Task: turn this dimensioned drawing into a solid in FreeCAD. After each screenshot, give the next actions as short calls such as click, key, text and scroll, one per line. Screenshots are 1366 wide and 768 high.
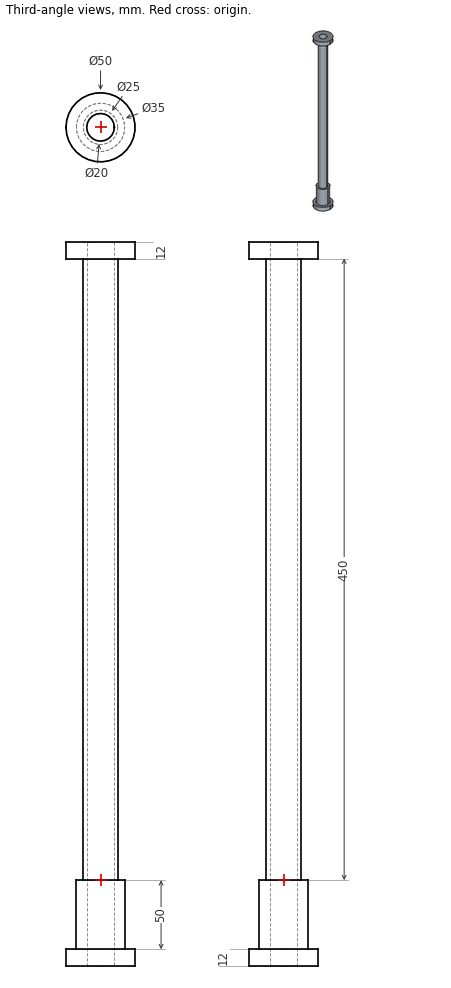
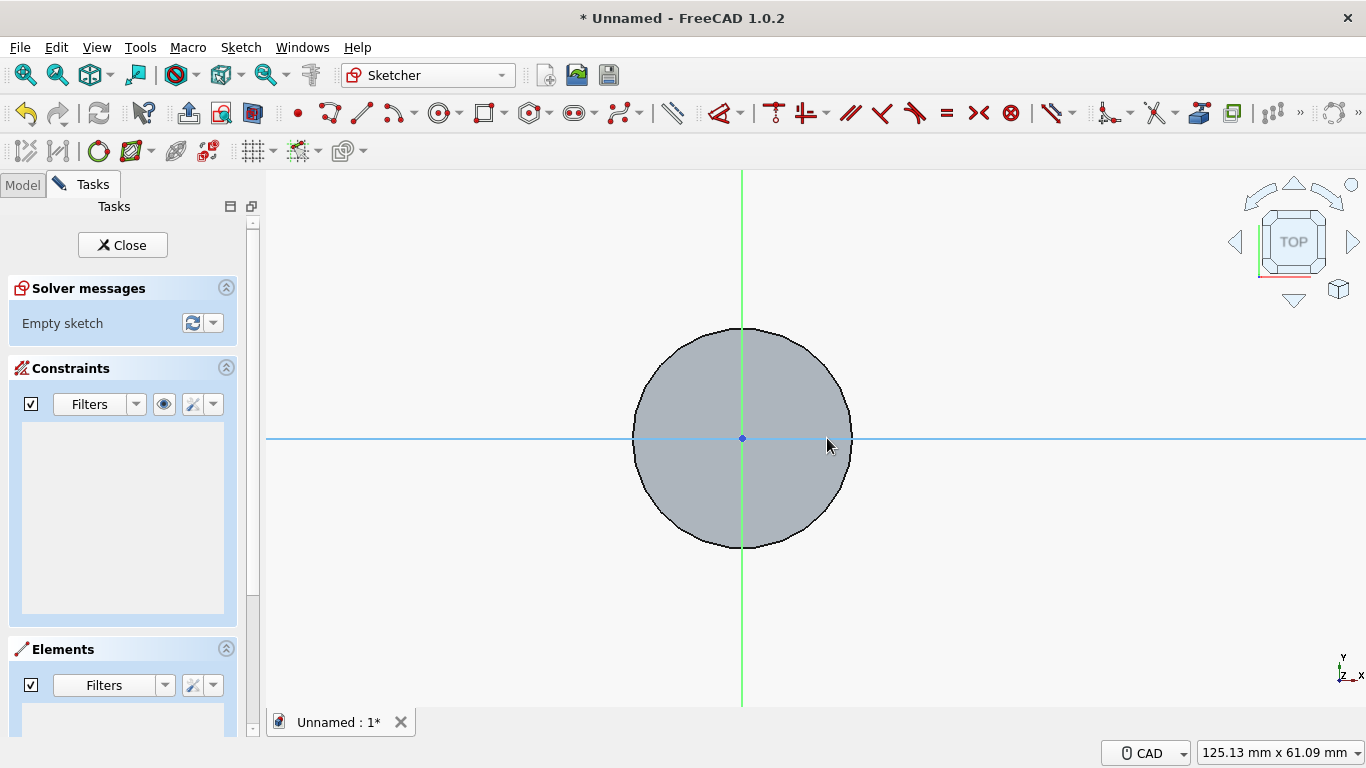
click(440, 114)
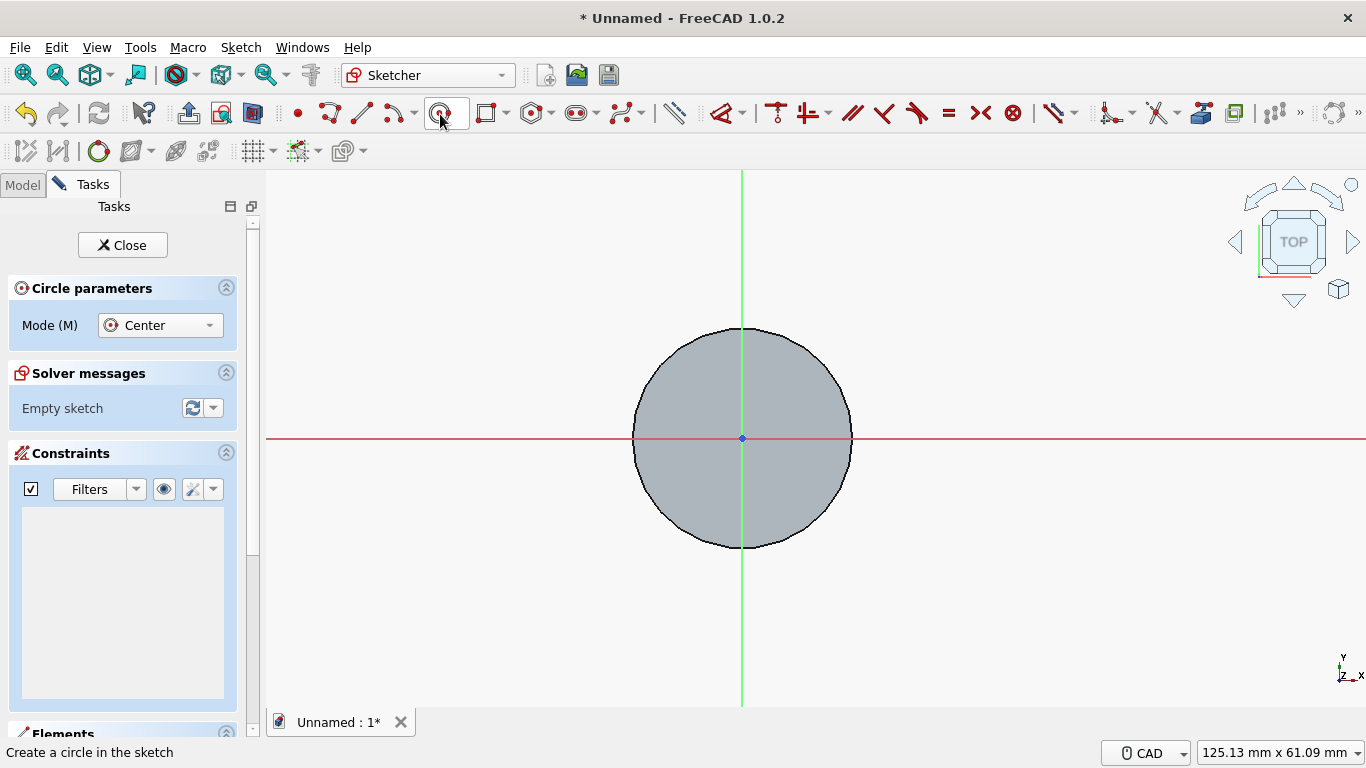
click(742, 438)
click(851, 330)
key(Escape)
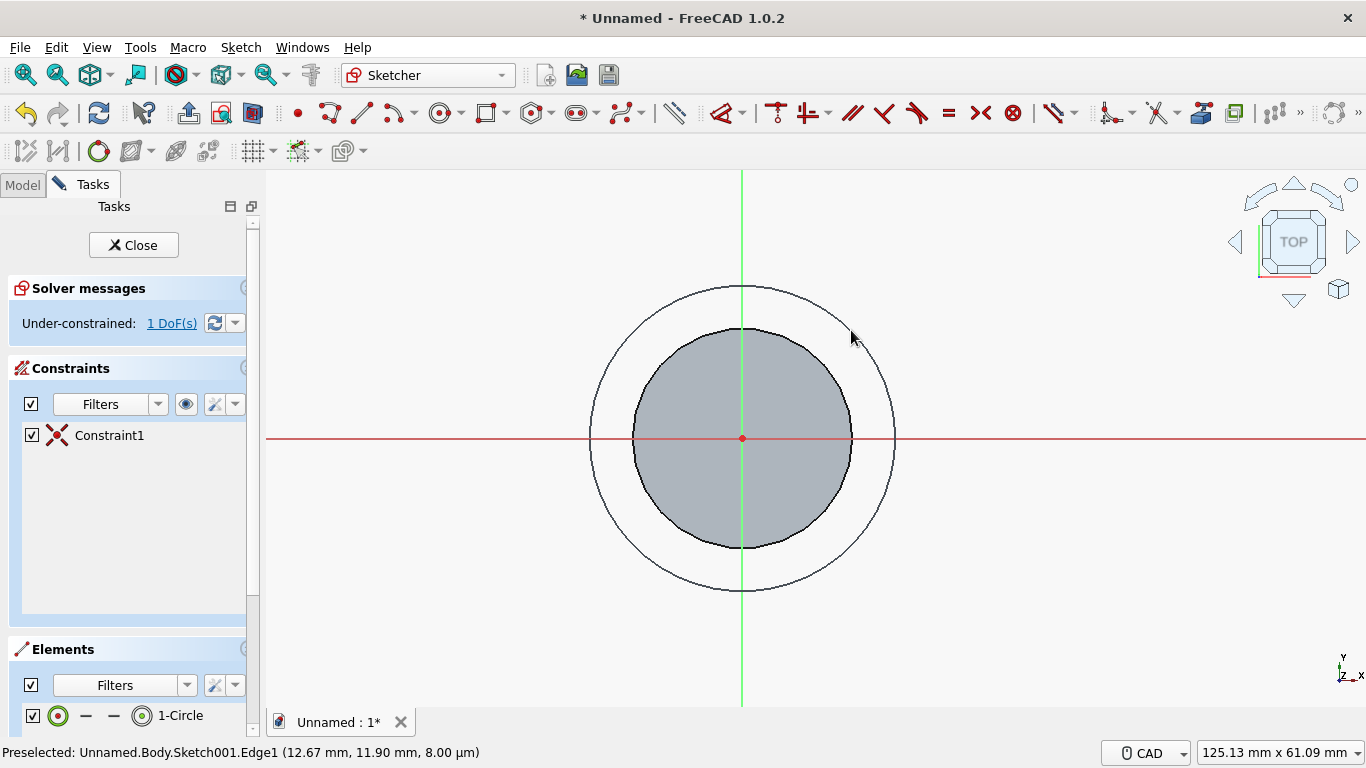
click(722, 114)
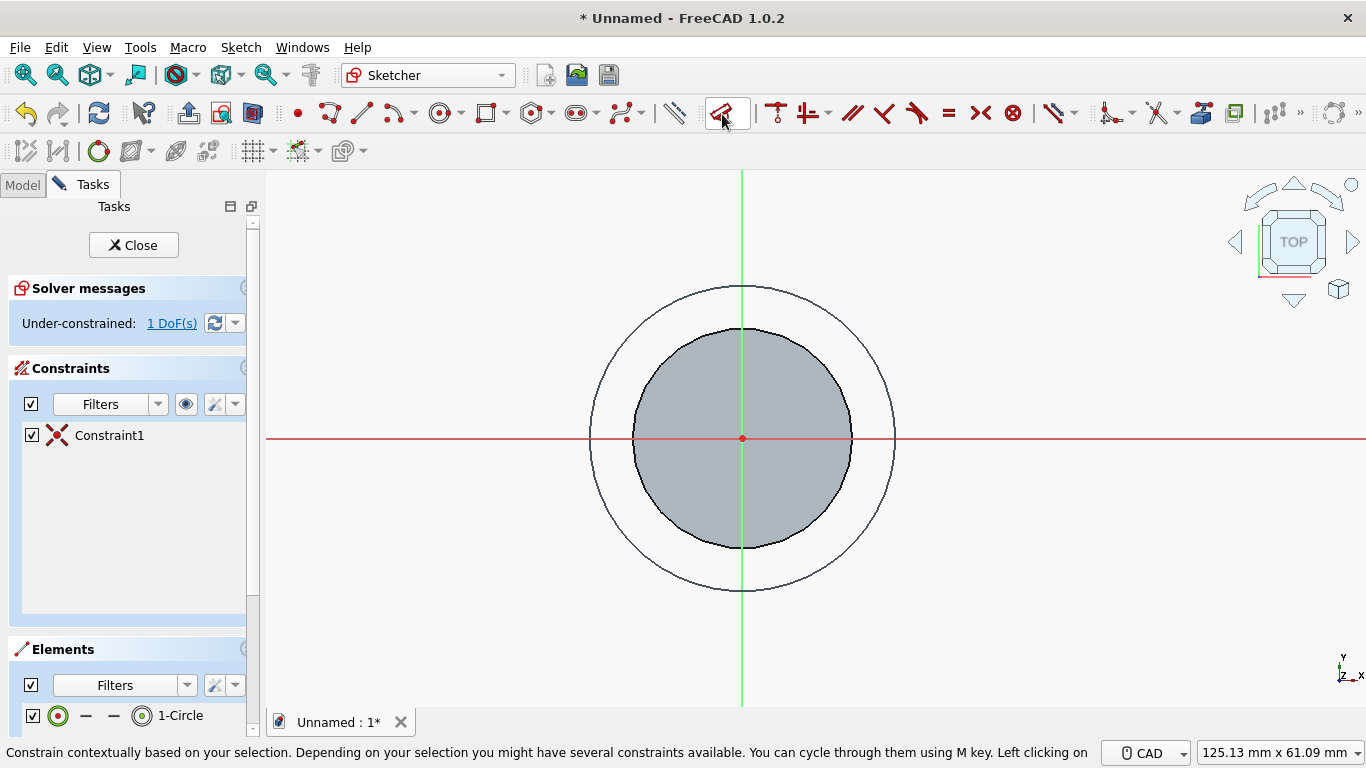
click(850, 330)
click(873, 307)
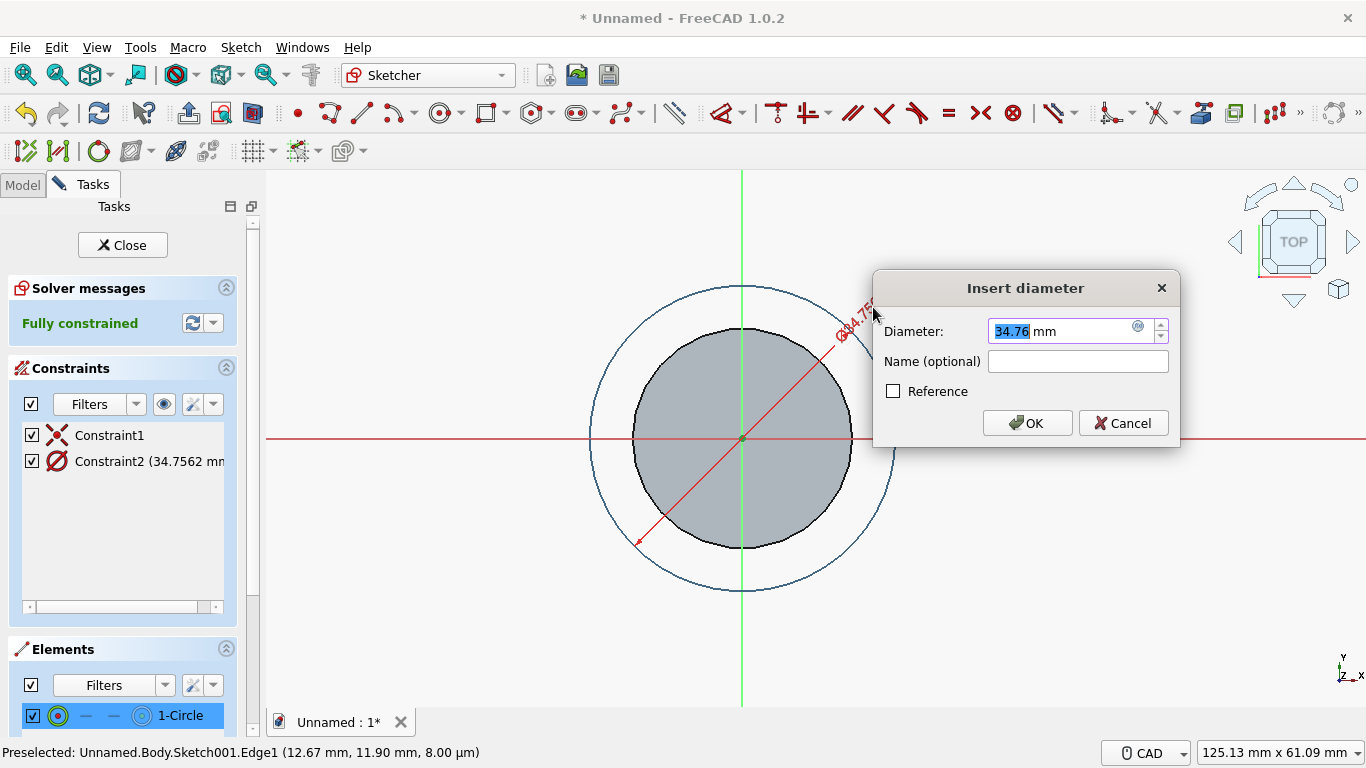
text(35)
key(Return)
key(Escape)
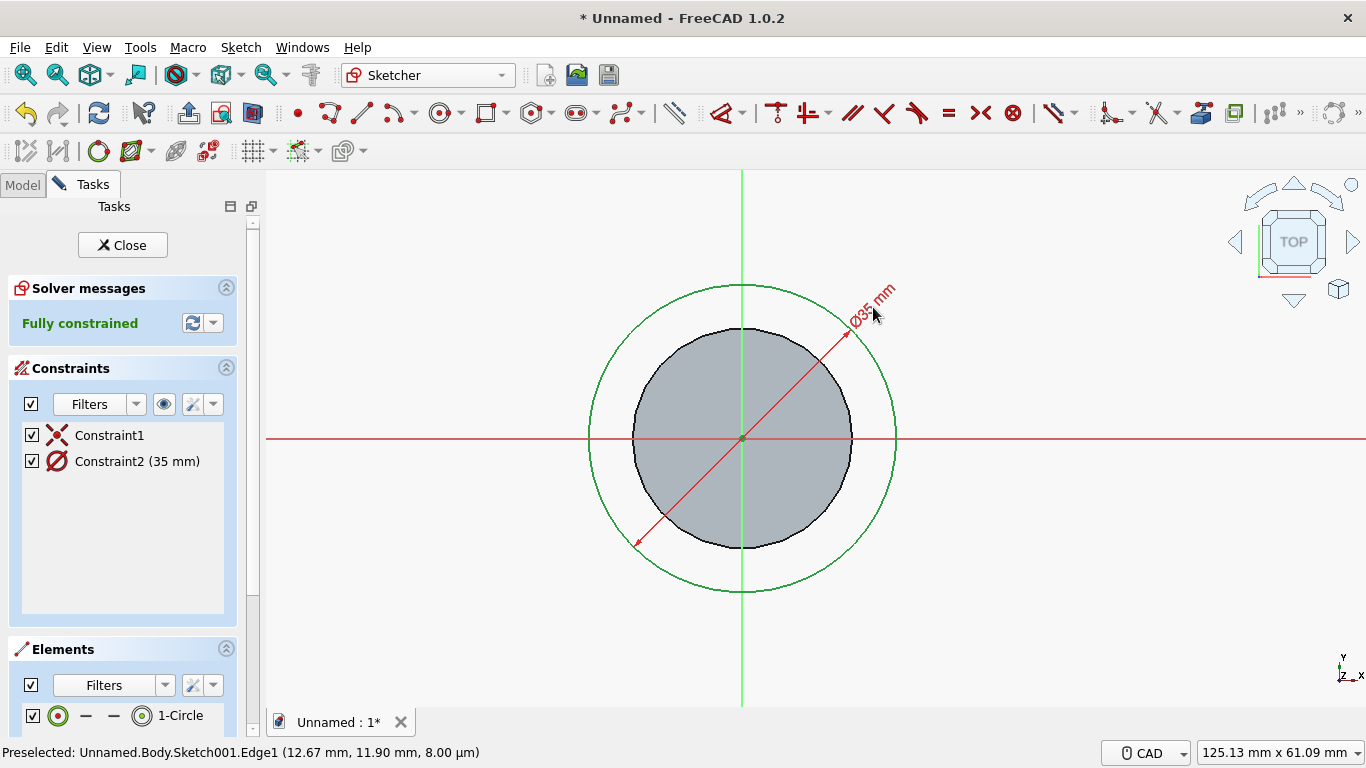
click(123, 245)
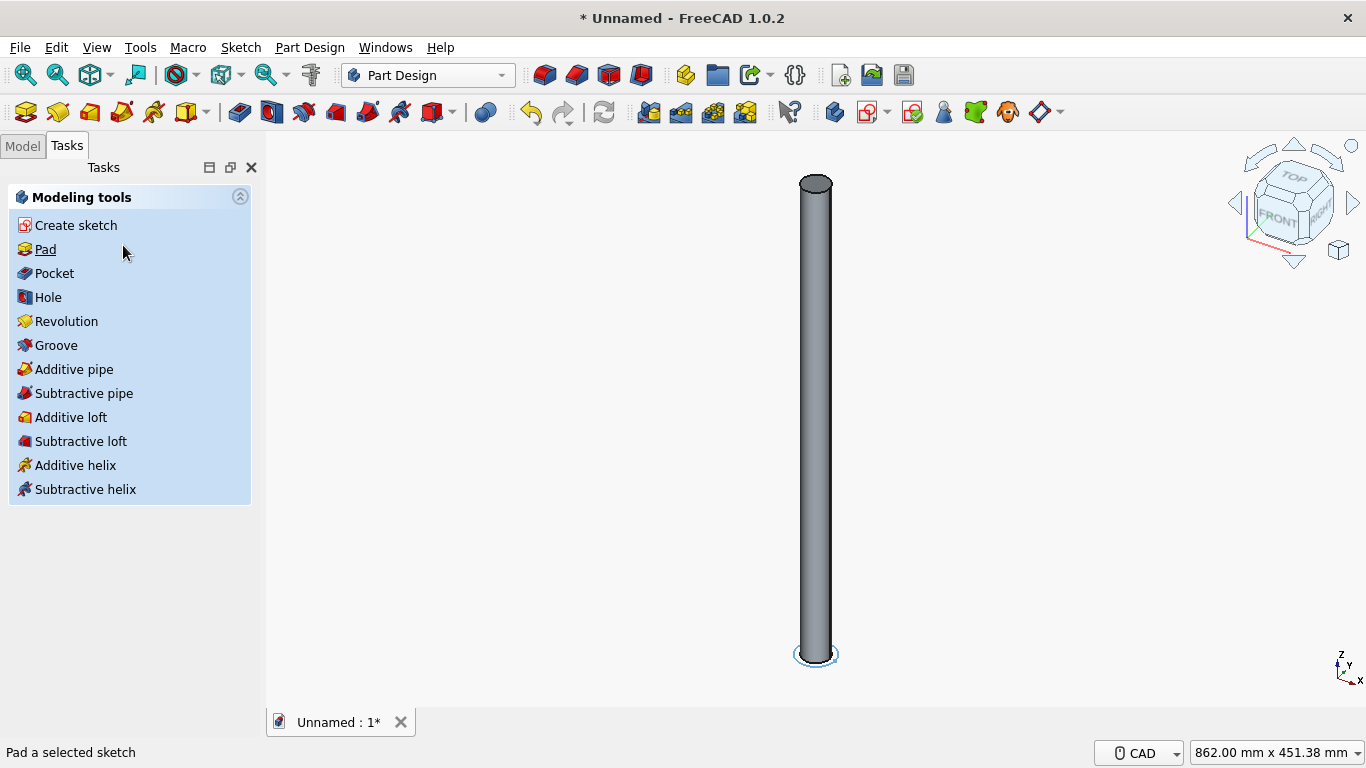
click(26, 112)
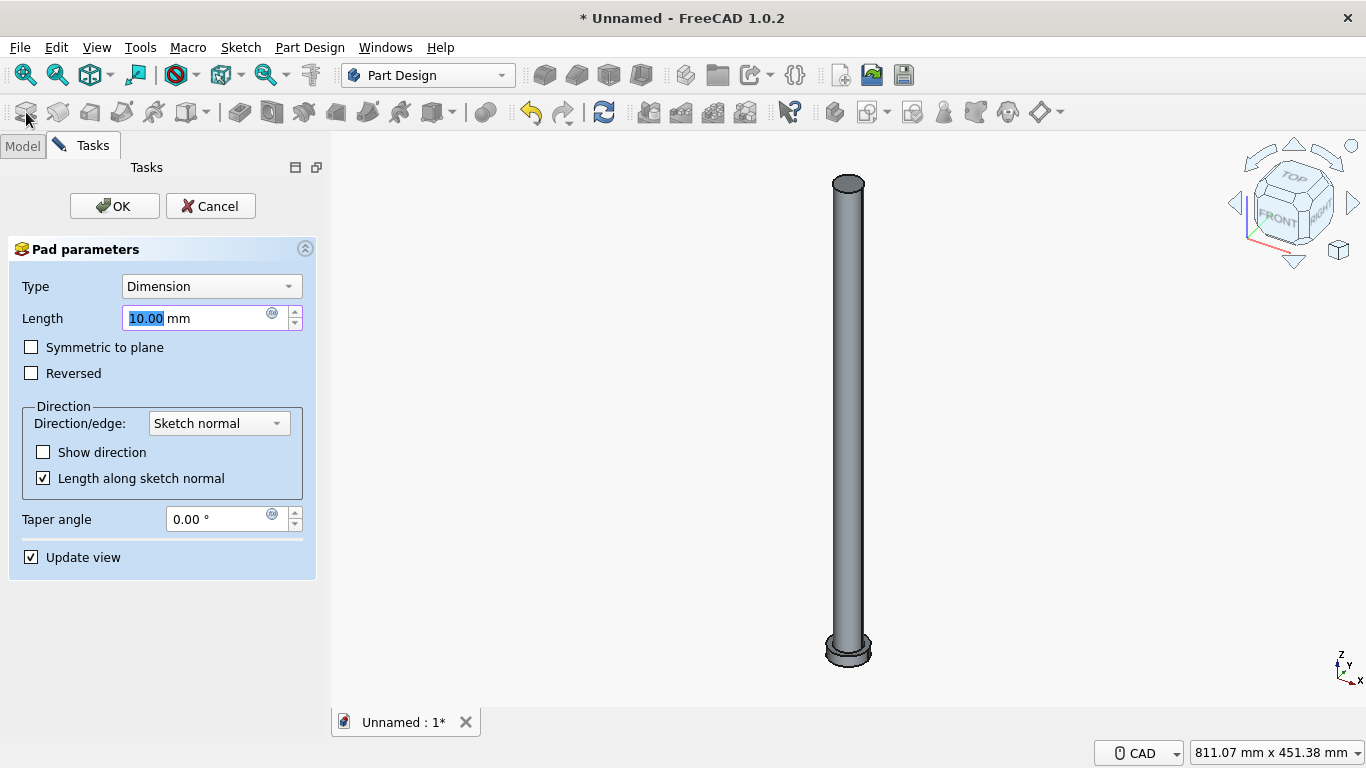
text(50)
key(Tab)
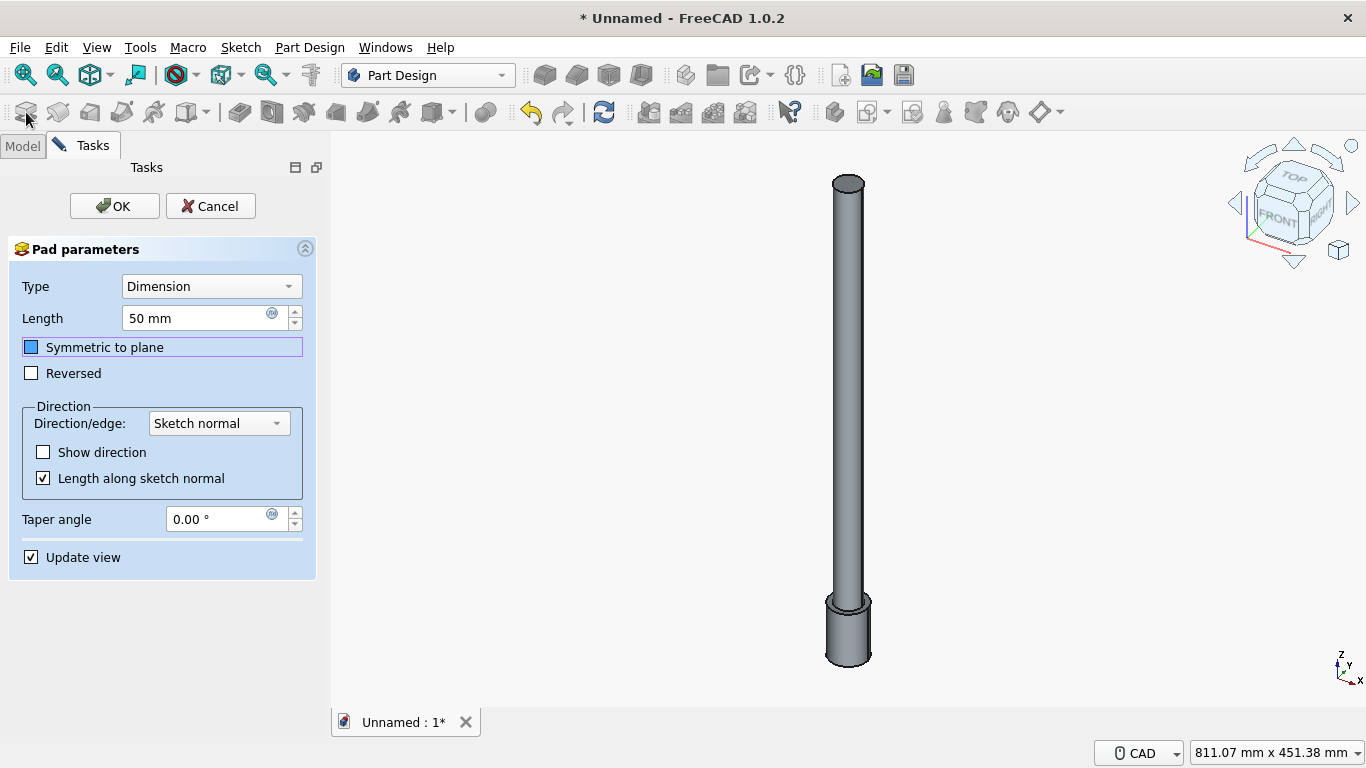
click(30, 373)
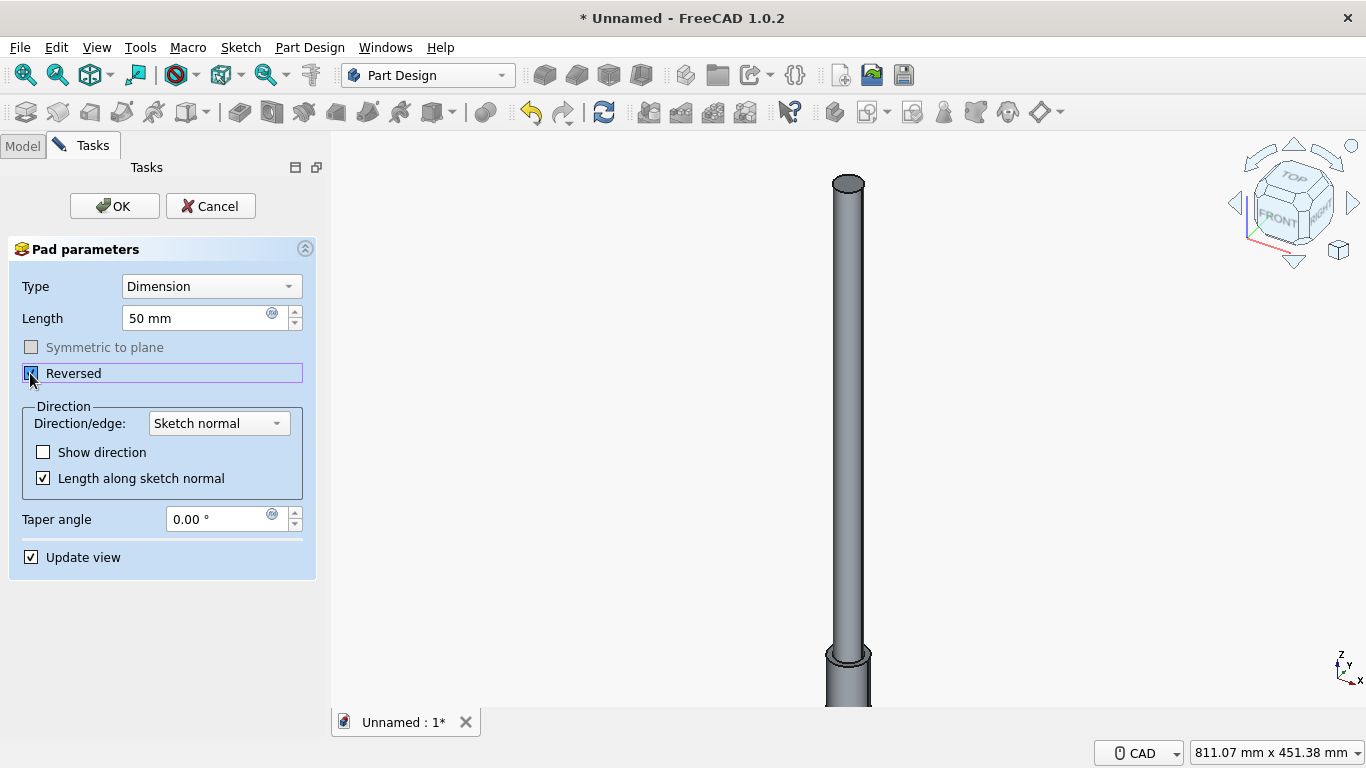
click(115, 206)